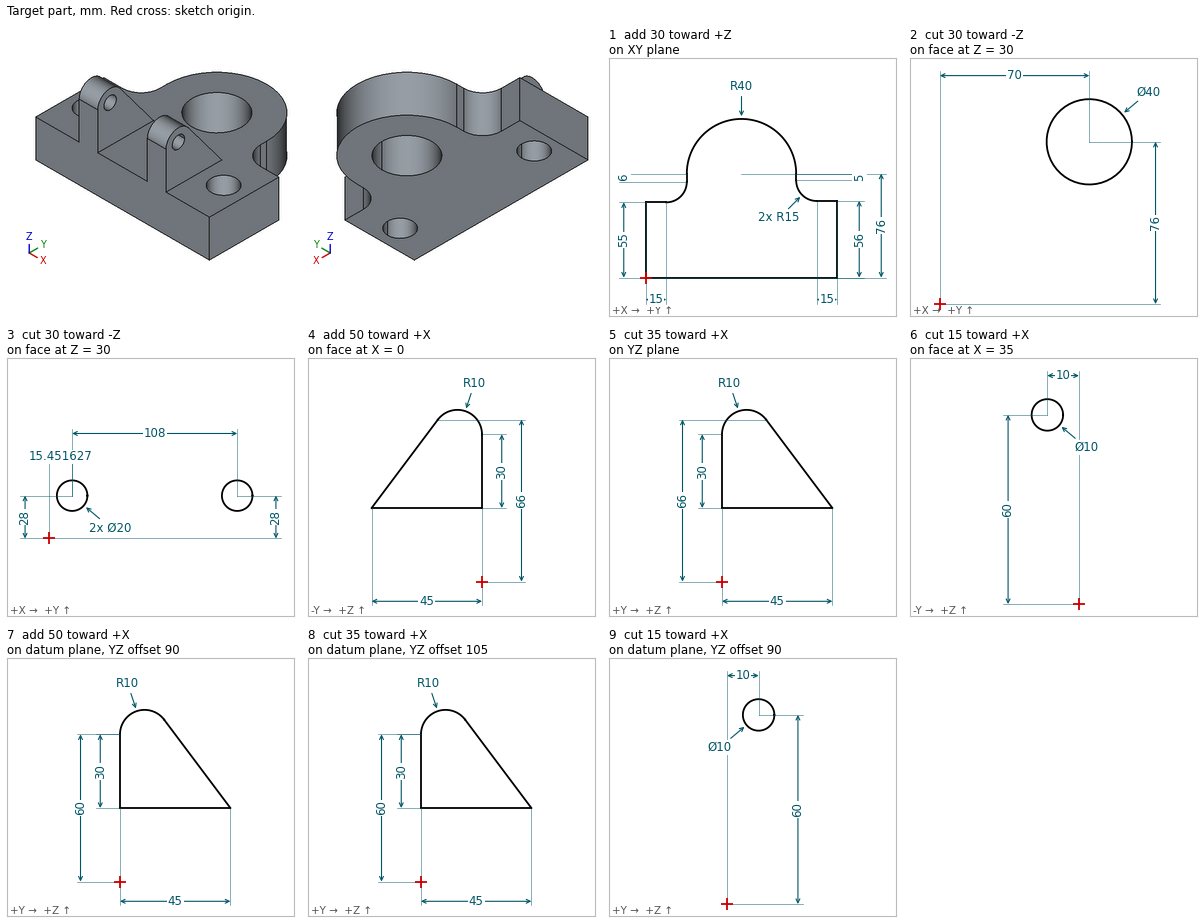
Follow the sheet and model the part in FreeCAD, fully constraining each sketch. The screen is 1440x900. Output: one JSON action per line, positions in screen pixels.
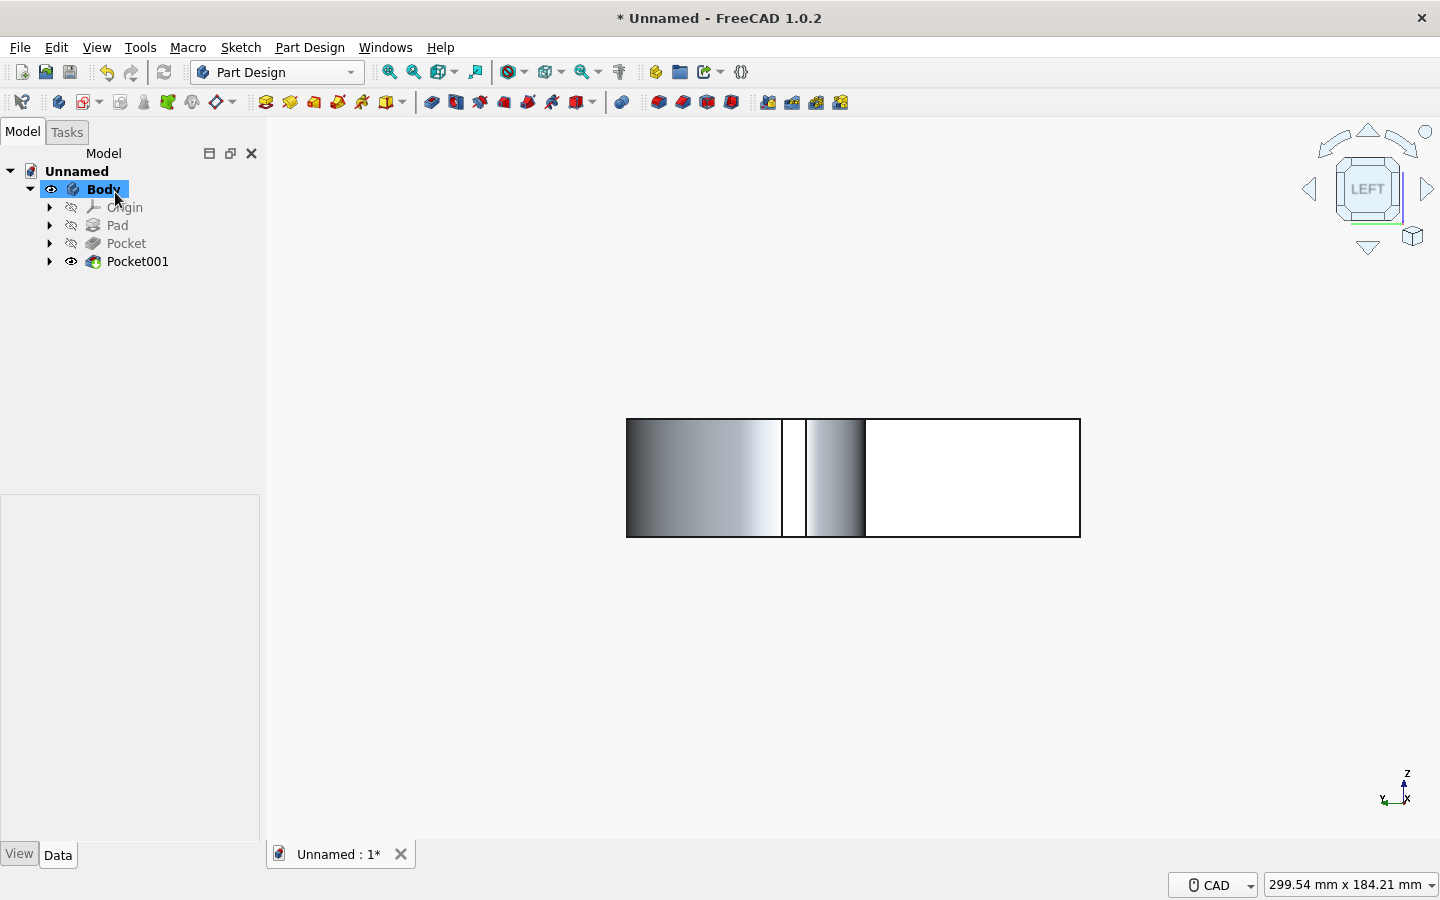
{"action": "key", "text": "v f"}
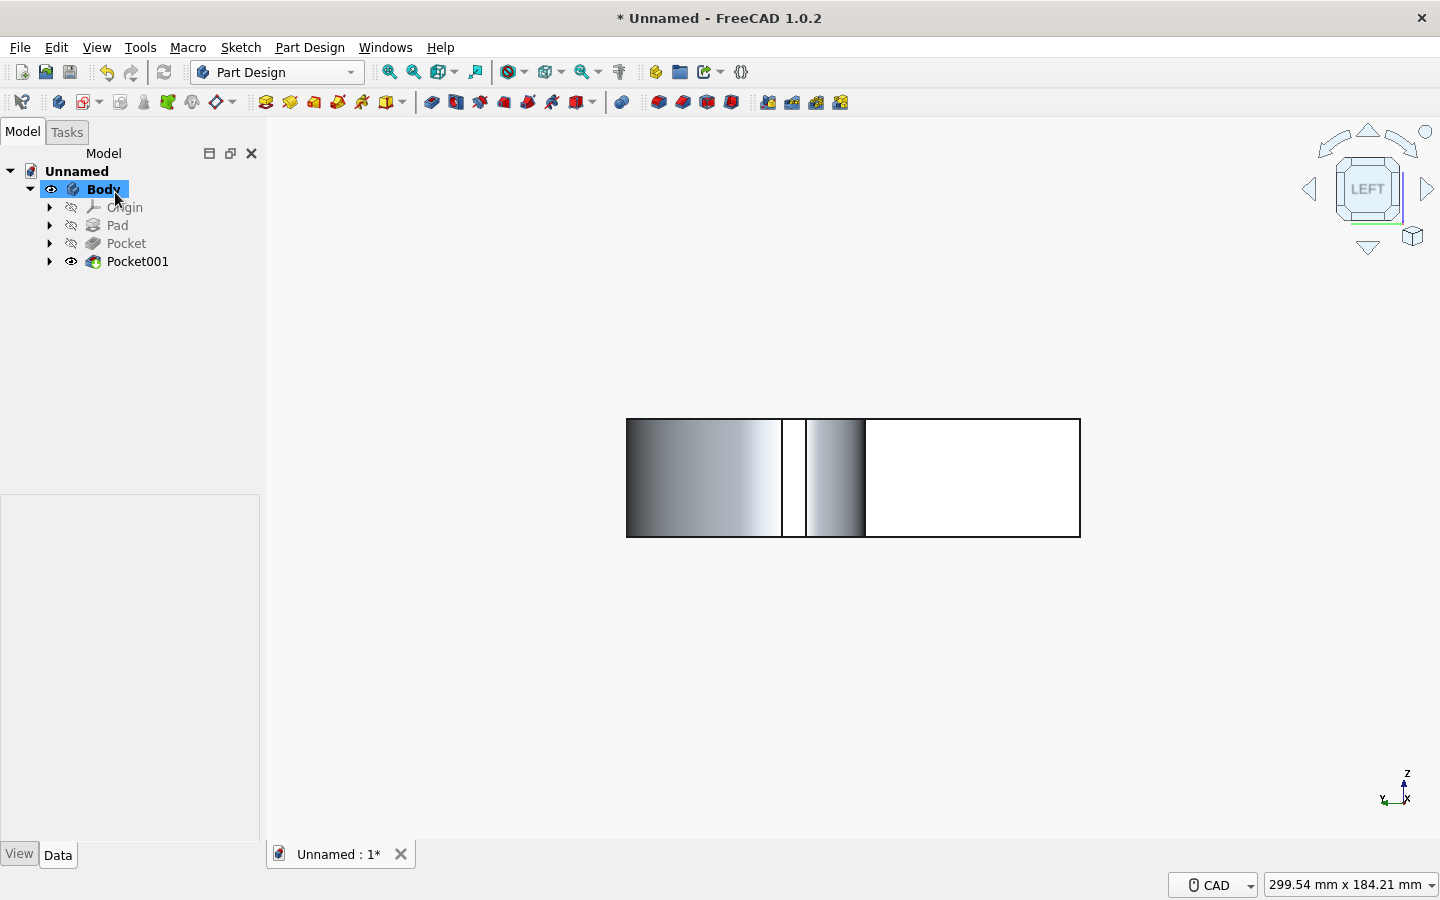
{"action": "left_click", "coordinate": [942, 477]}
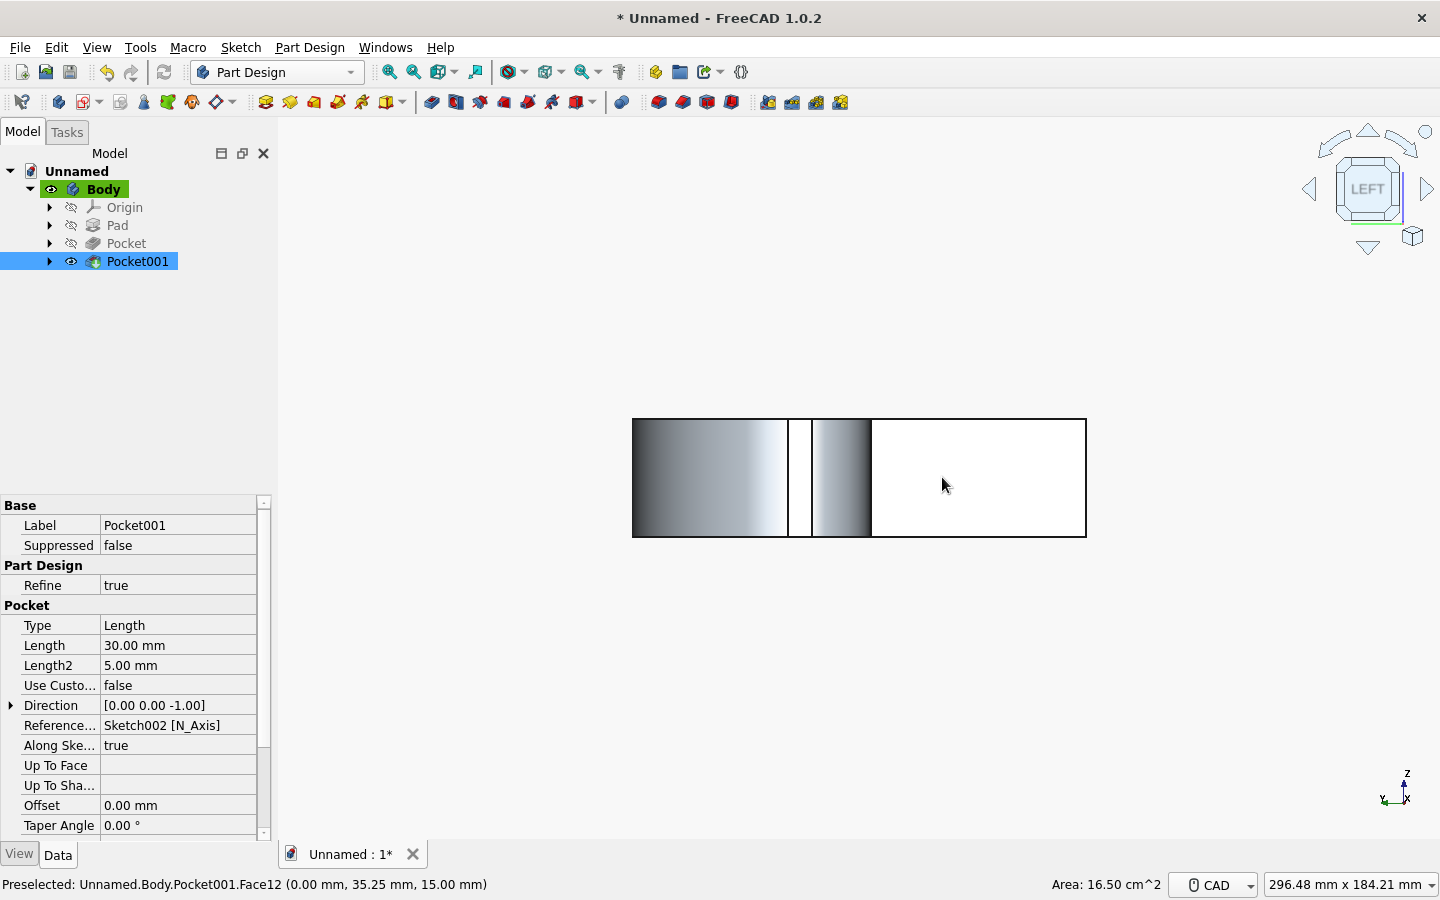
{"action": "left_click", "coordinate": [84, 102]}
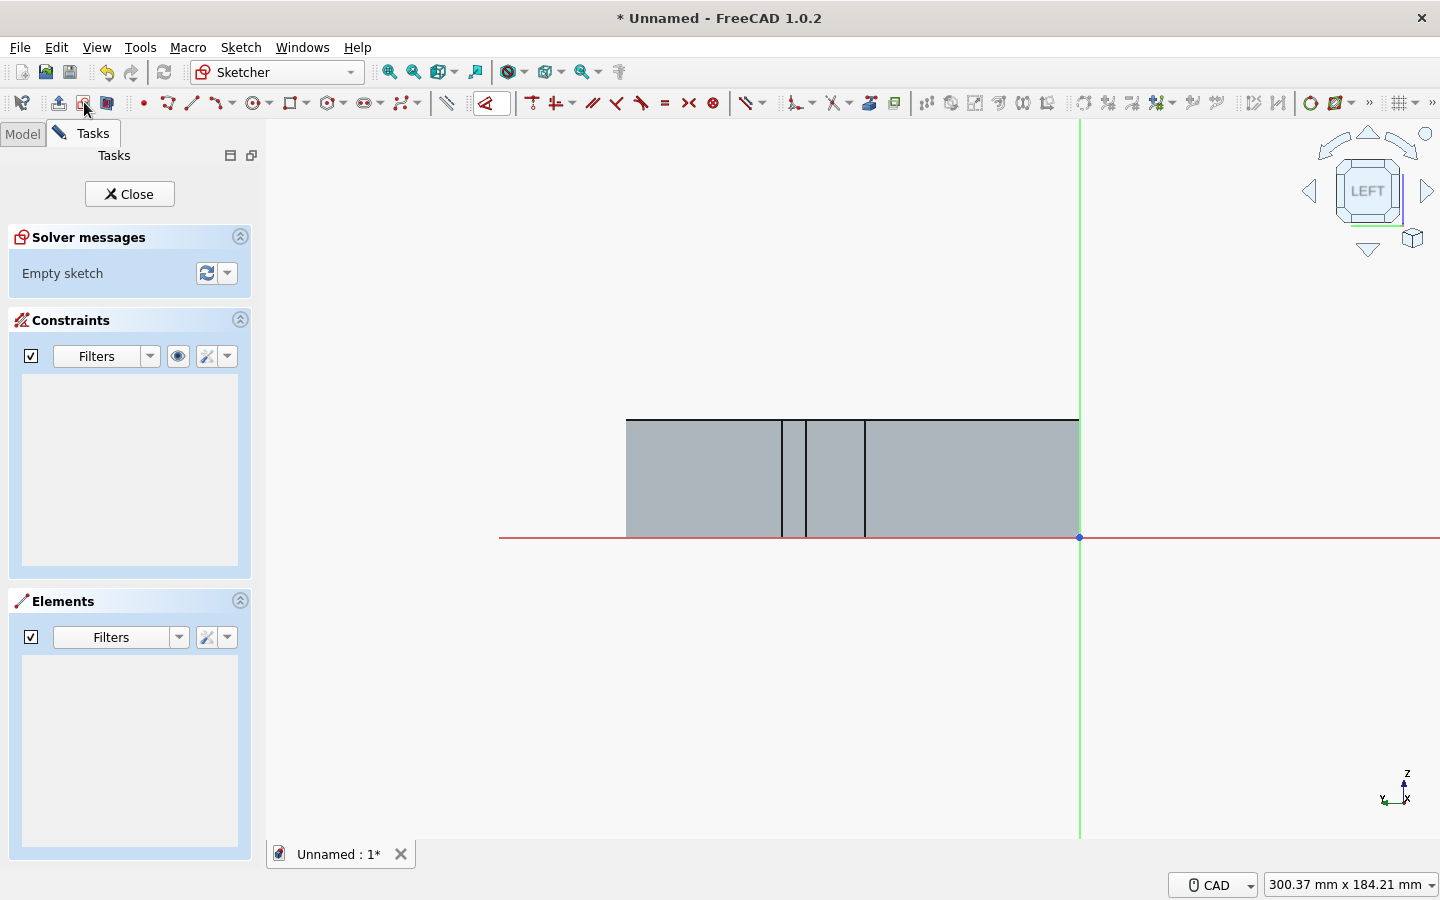
{"action": "scroll", "coordinate": [1243, 308], "scroll_direction": "up", "scroll_amount": 3}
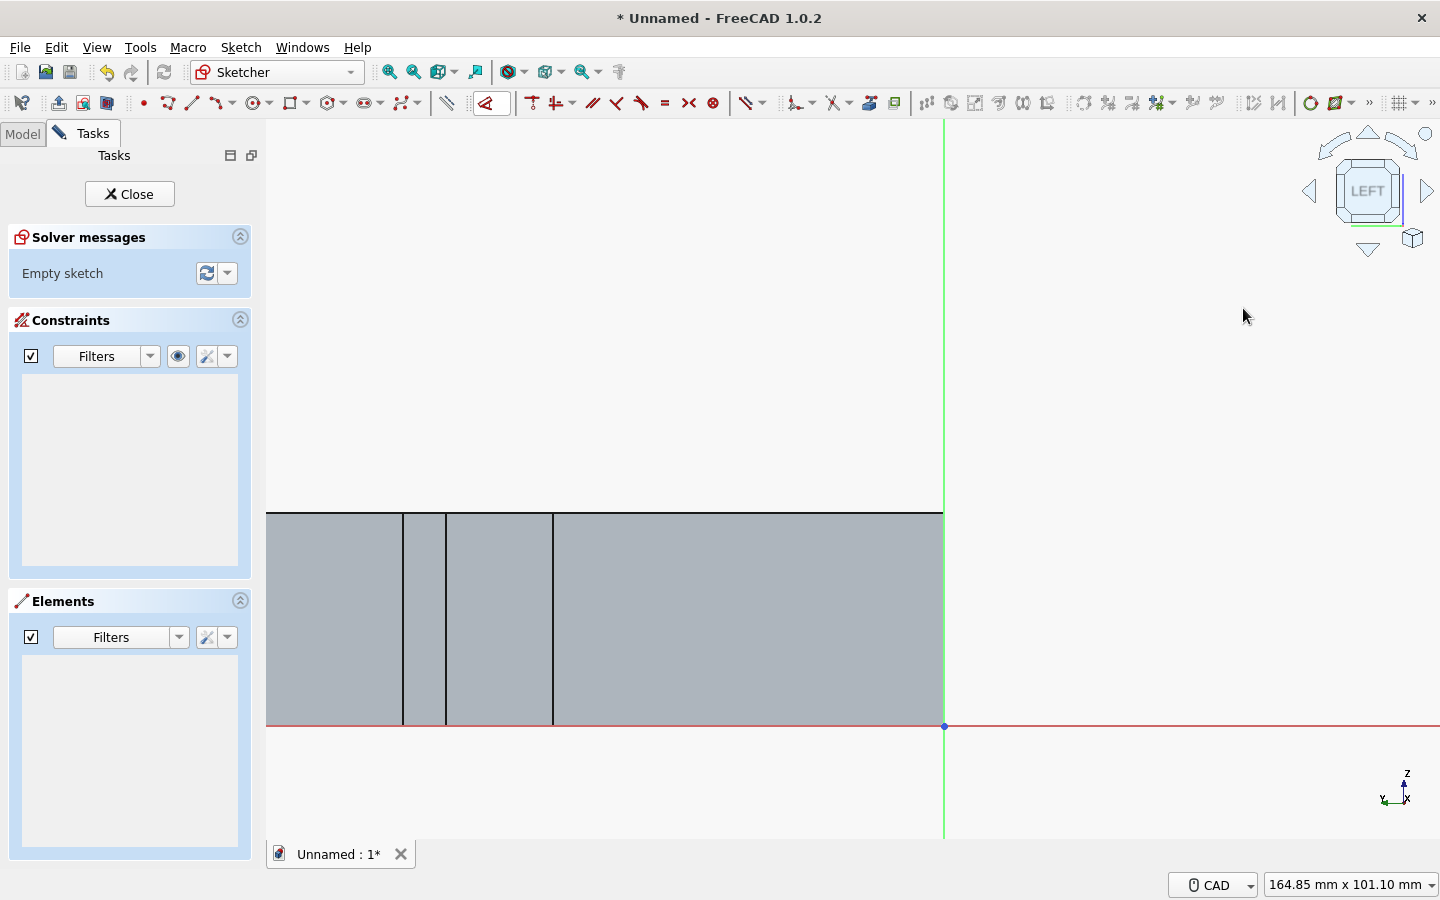
{"action": "left_click", "coordinate": [168, 104]}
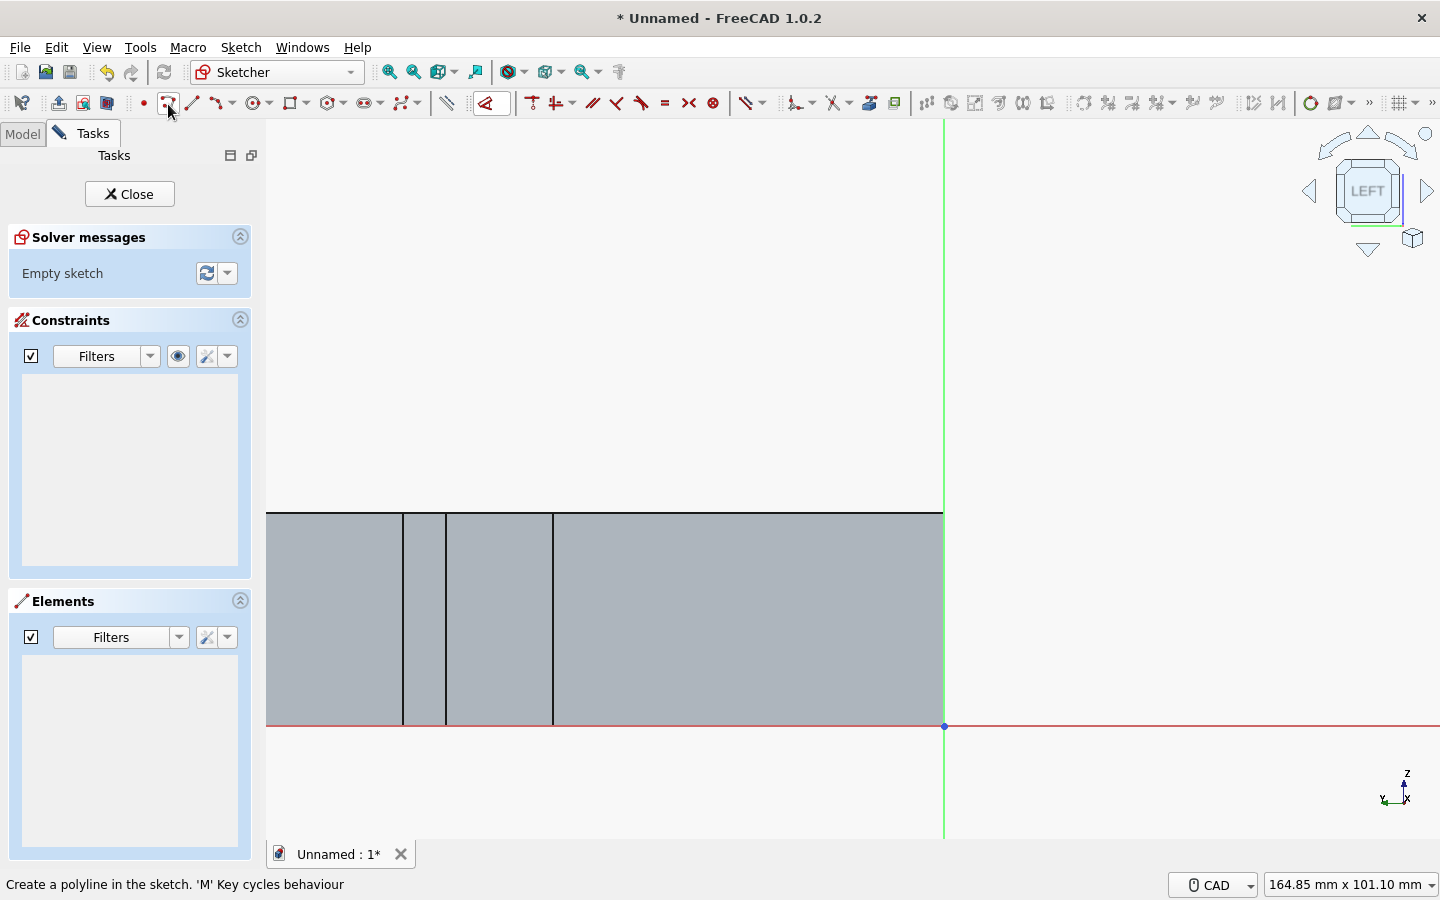
{"action": "left_click", "coordinate": [816, 256]}
{"action": "left_click", "coordinate": [624, 513]}
{"action": "left_click", "coordinate": [944, 513]}
{"action": "left_click", "coordinate": [935, 299]}
{"action": "right_click", "coordinate": [935, 299]}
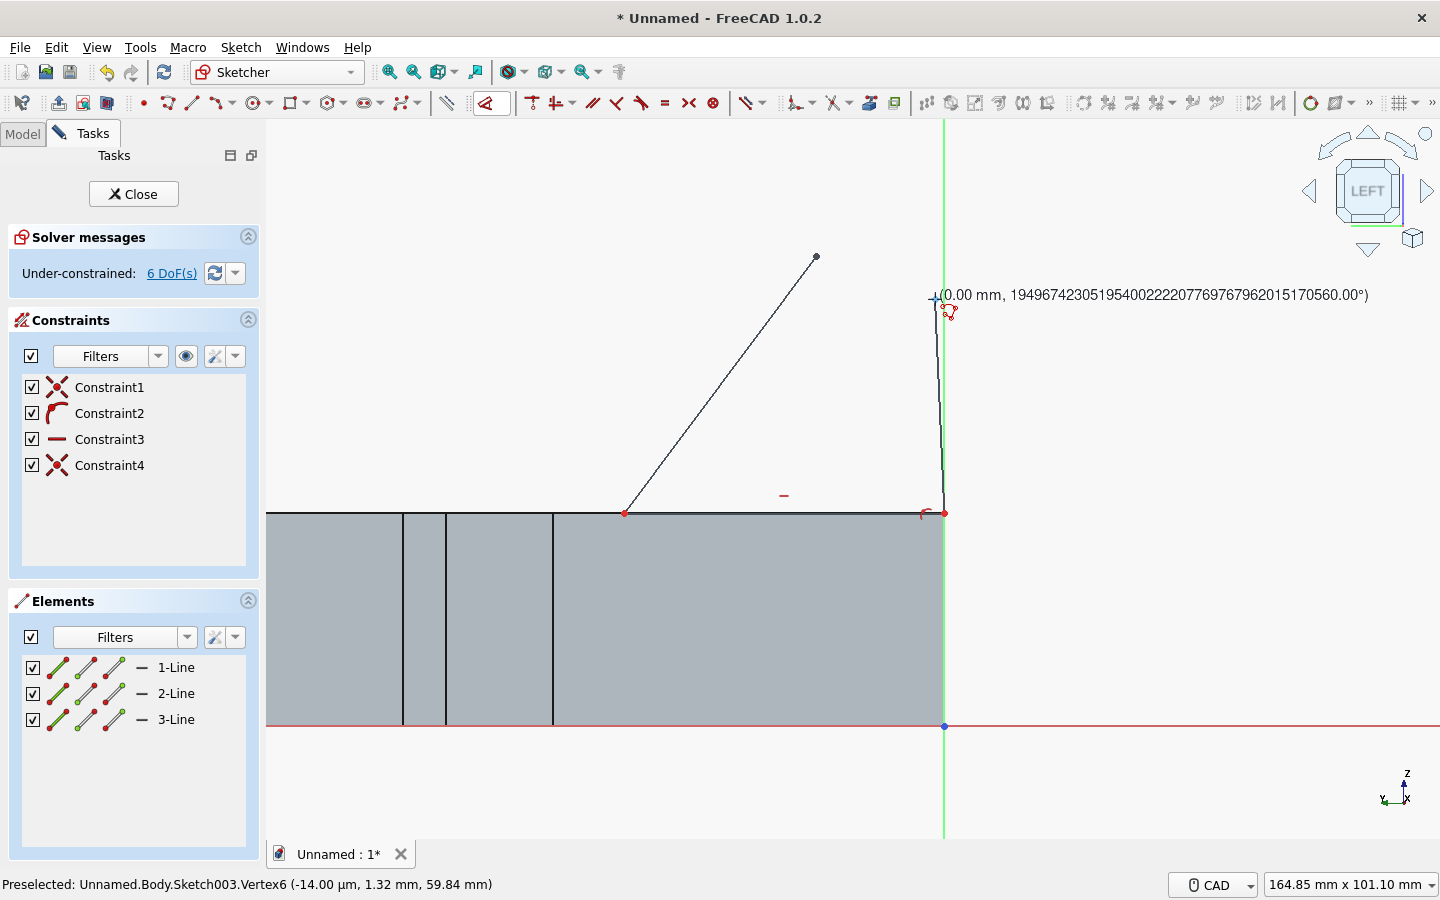
{"action": "key", "text": "g 3 a"}